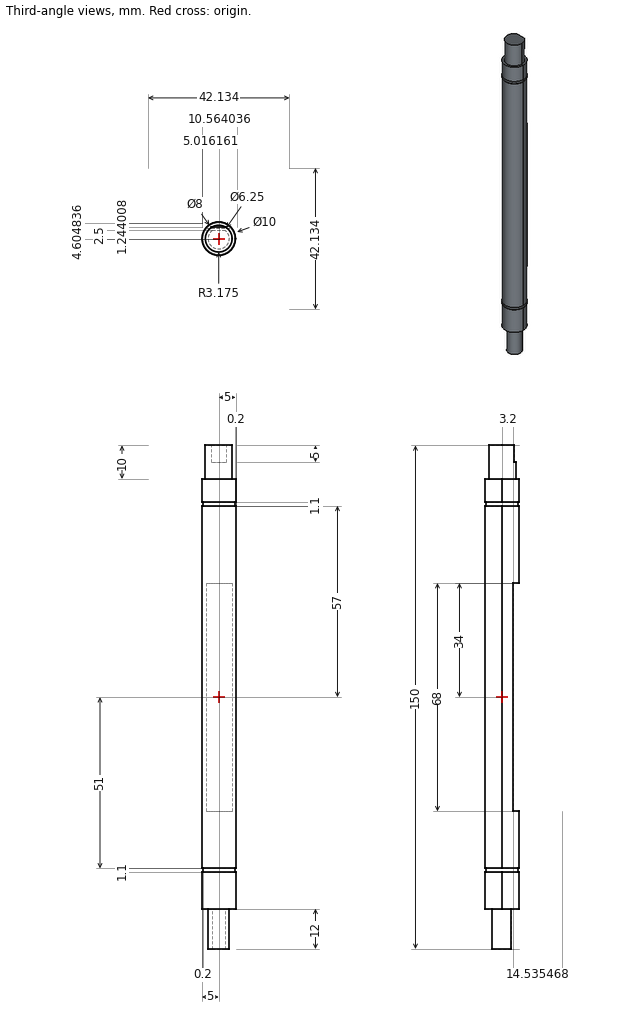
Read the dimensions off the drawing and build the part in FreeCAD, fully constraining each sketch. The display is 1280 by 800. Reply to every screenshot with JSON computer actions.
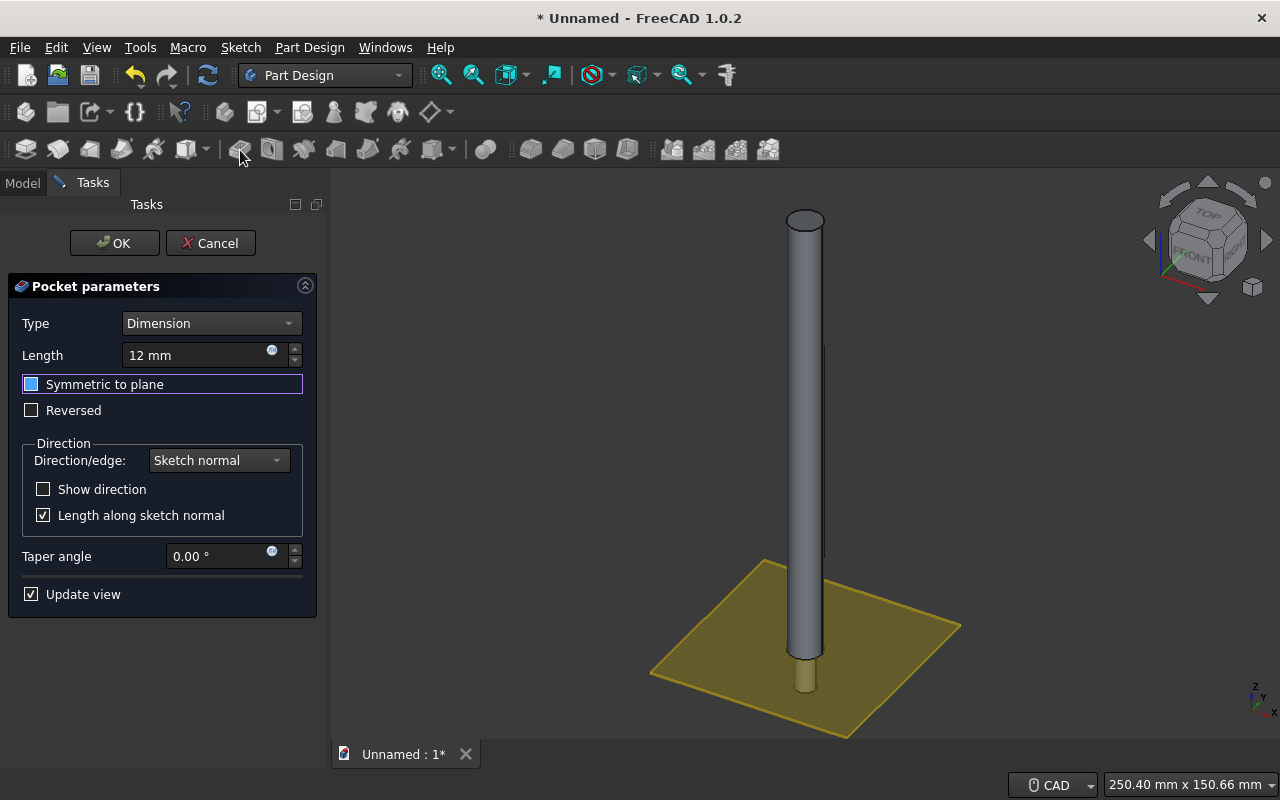
{"action": "left_click", "coordinate": [115, 243]}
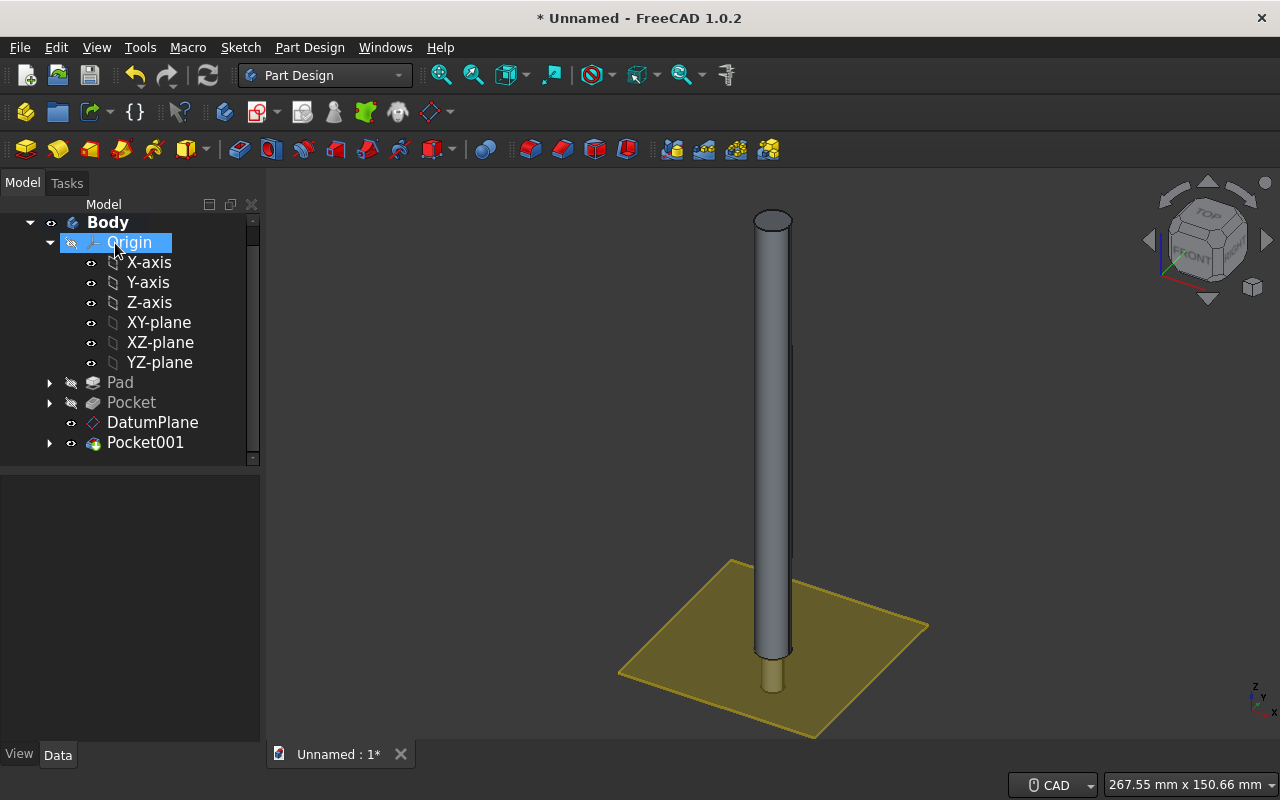
{"action": "left_click", "coordinate": [116, 423]}
{"action": "key", "text": "space"}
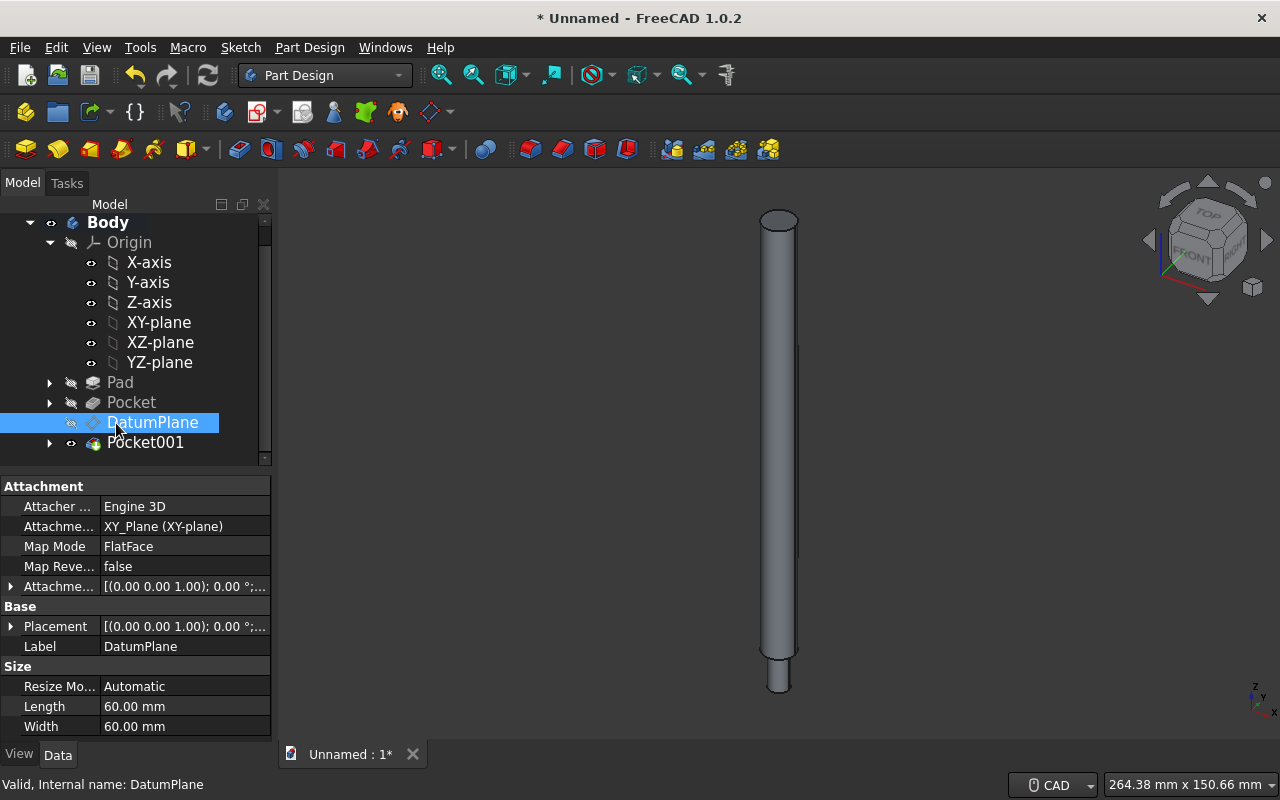
{"action": "key", "text": "5"}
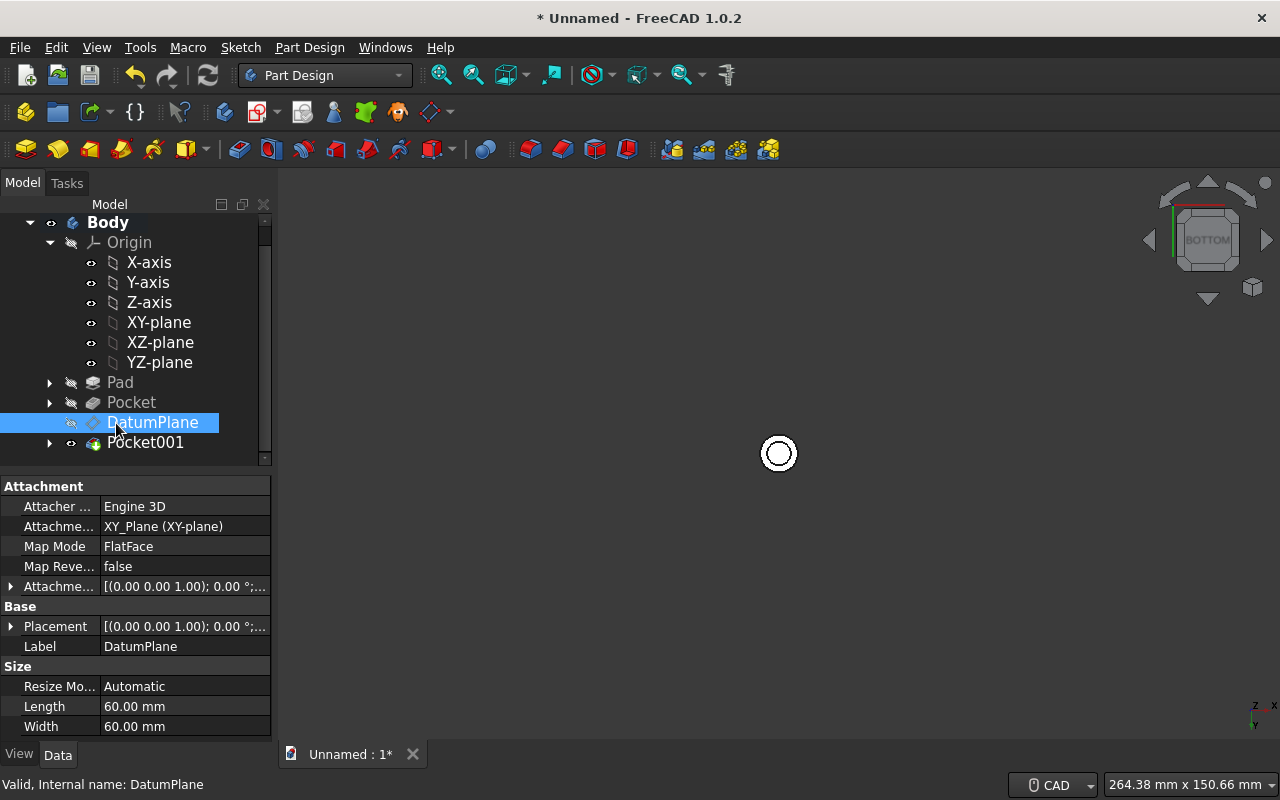
{"action": "left_click", "coordinate": [442, 76]}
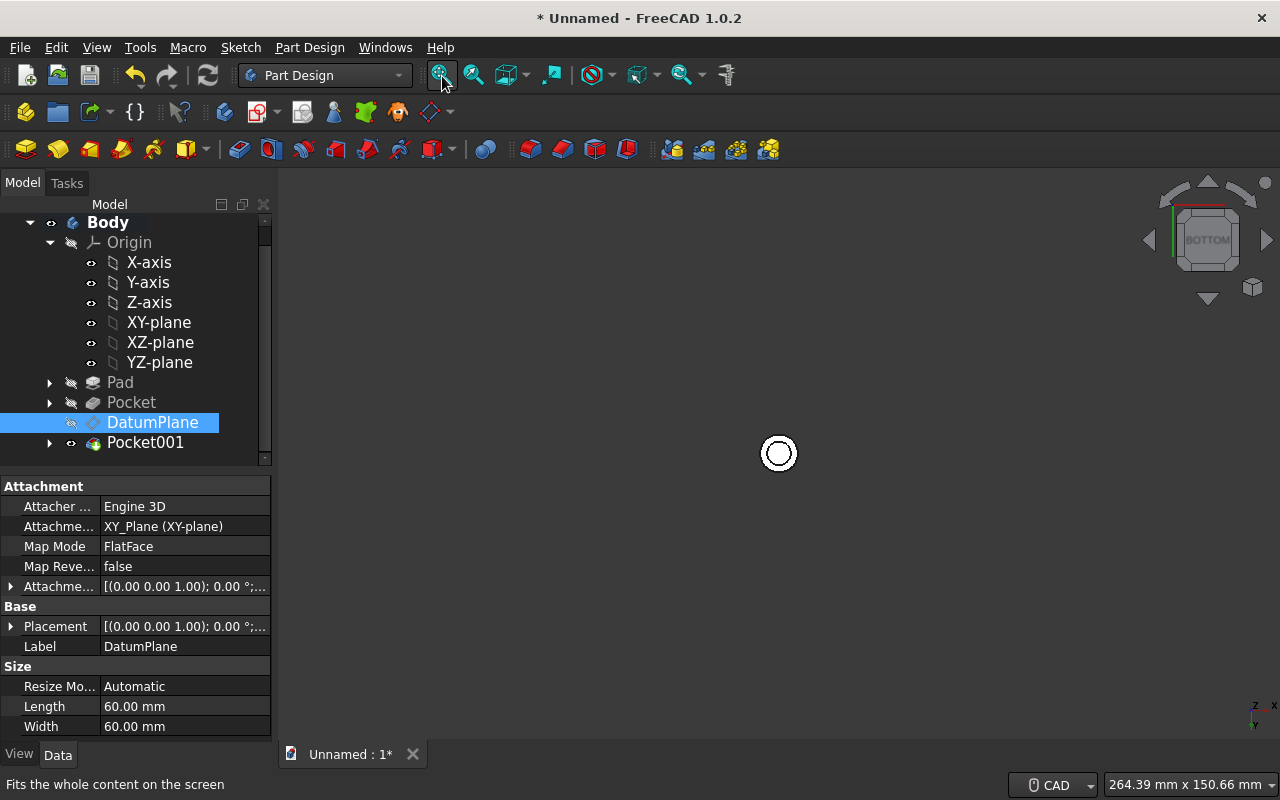
{"action": "left_click", "coordinate": [779, 452]}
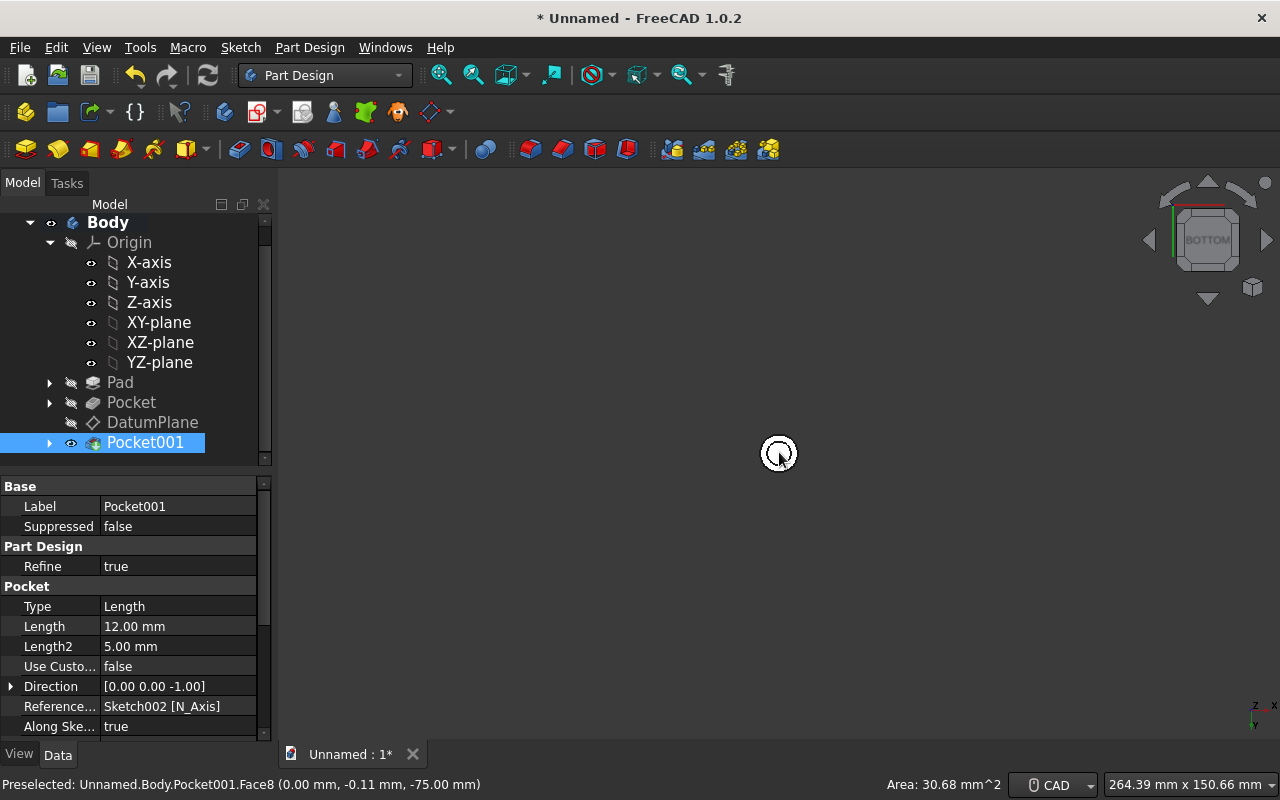
{"action": "left_click", "coordinate": [258, 112]}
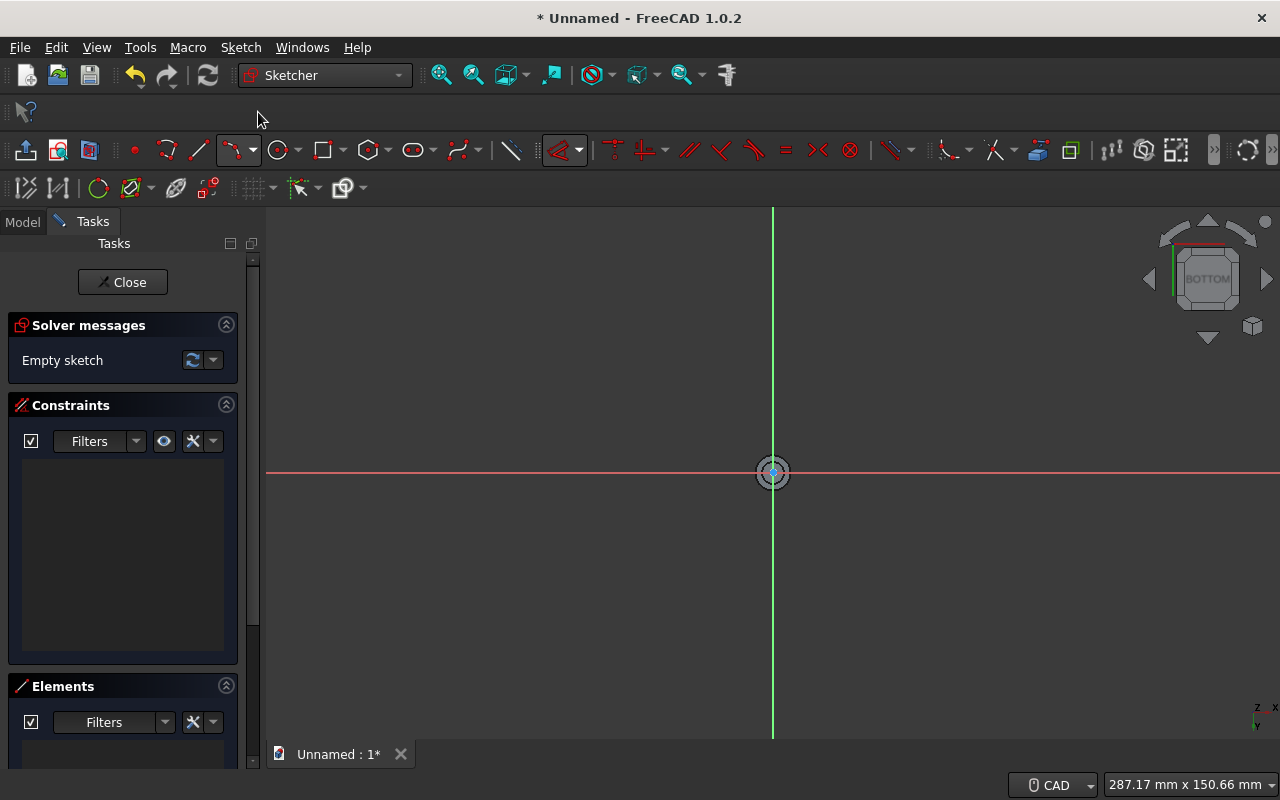
{"action": "scroll", "coordinate": [829, 473], "scroll_direction": "up", "scroll_amount": 4}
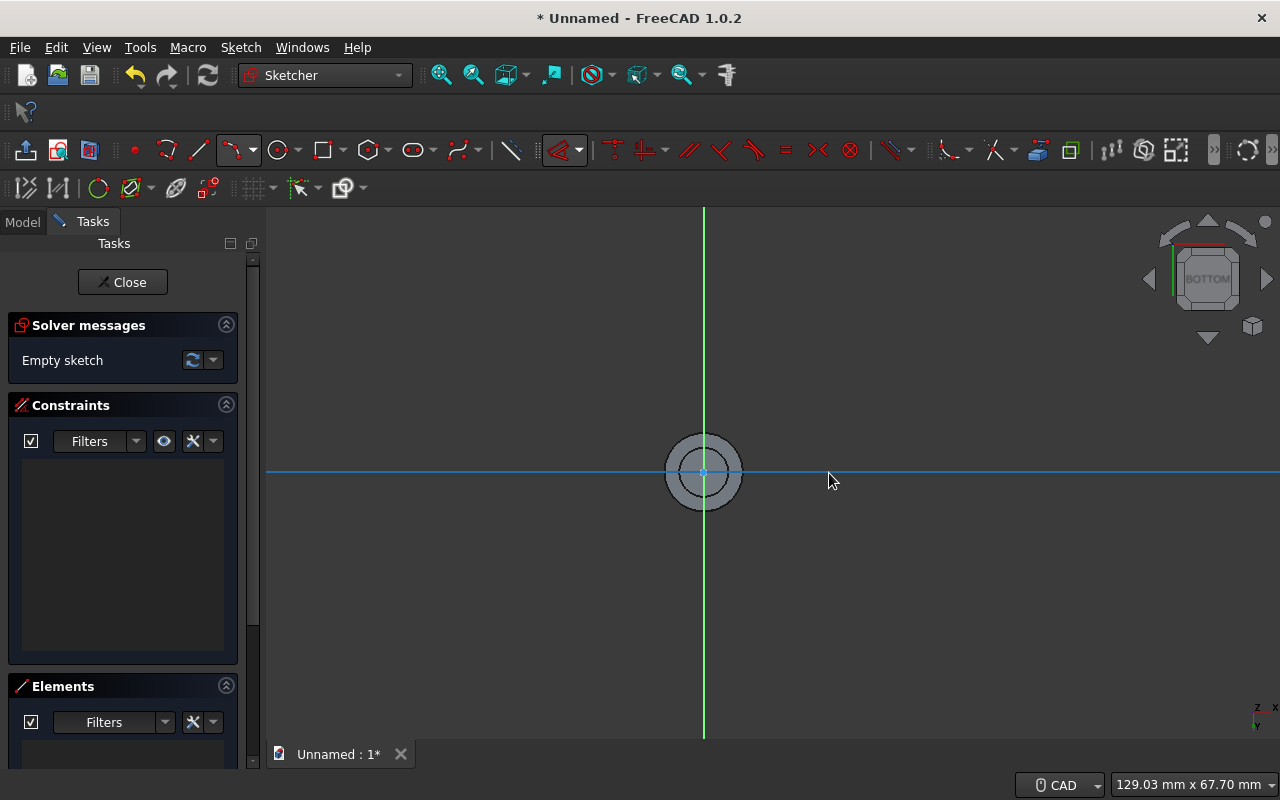
{"action": "left_click", "coordinate": [346, 150]}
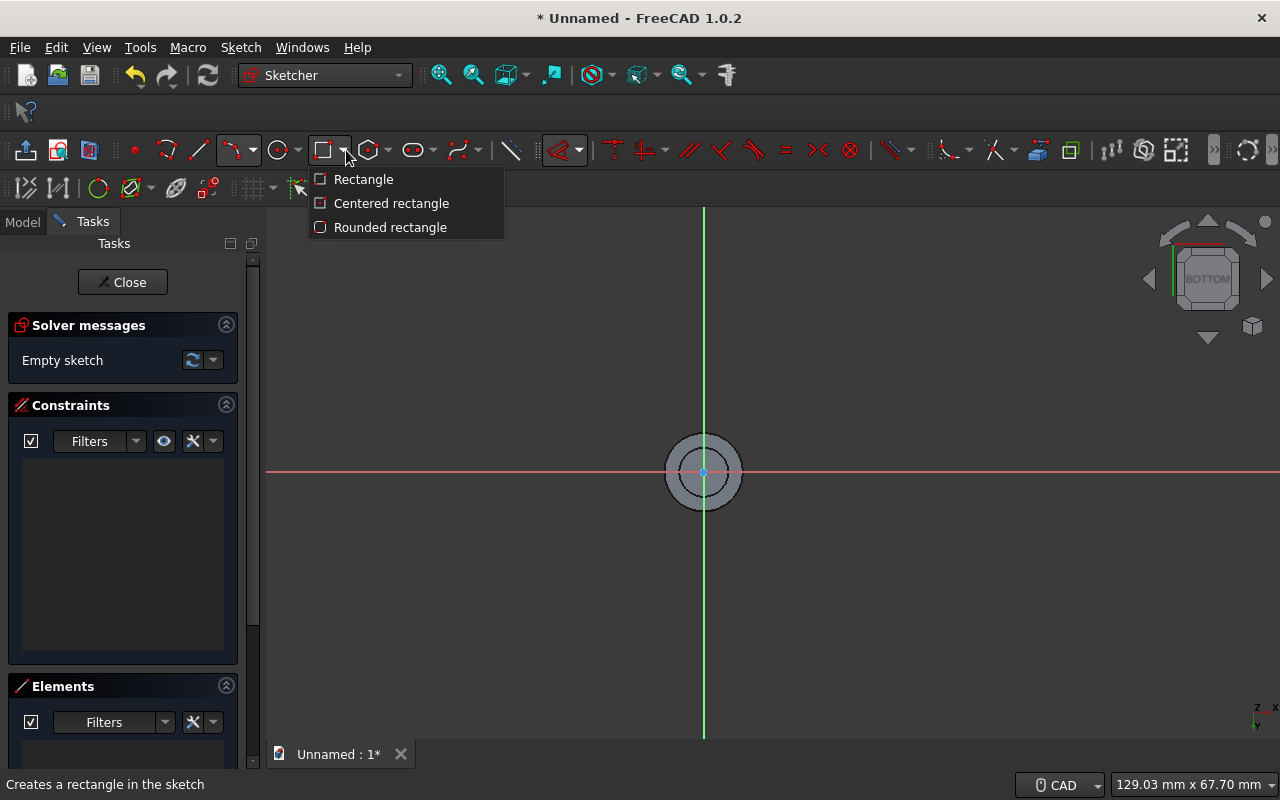
{"action": "left_click", "coordinate": [406, 203]}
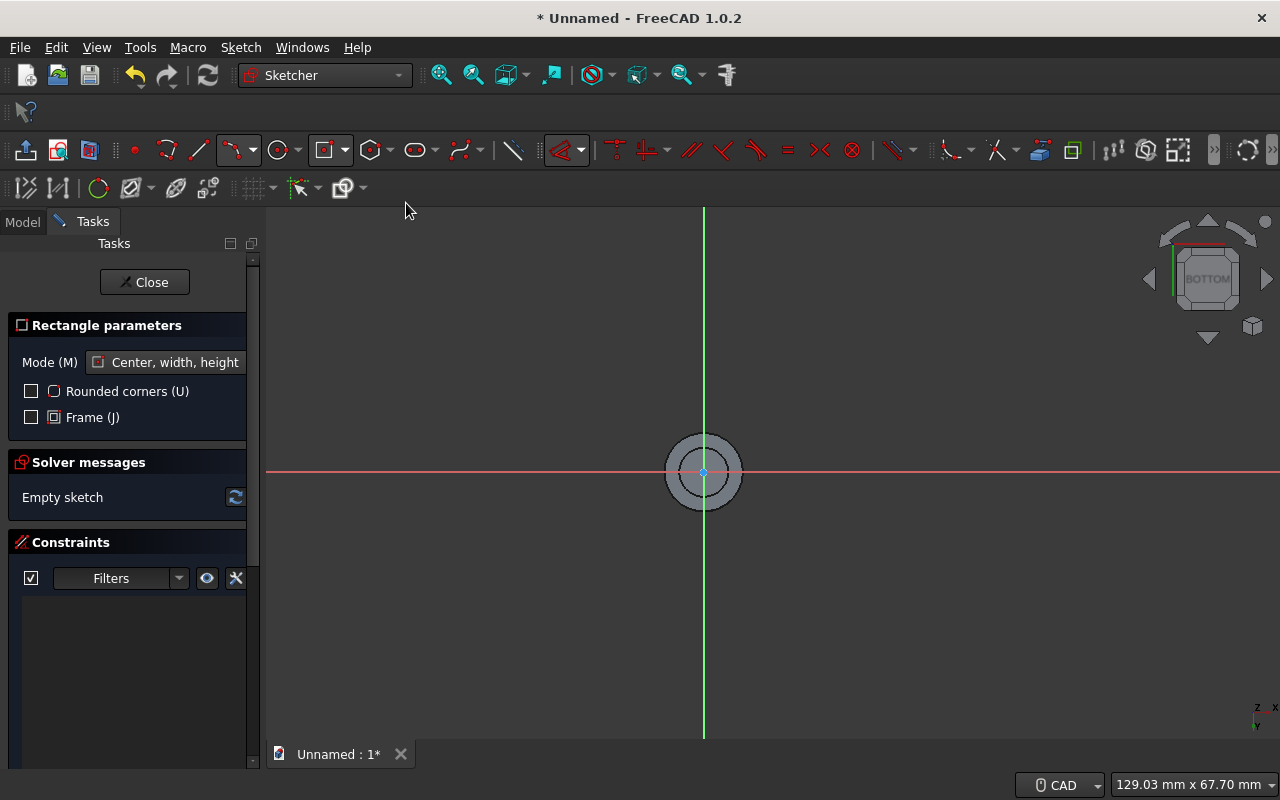
{"action": "left_click", "coordinate": [704, 472]}
{"action": "left_click", "coordinate": [869, 307]}